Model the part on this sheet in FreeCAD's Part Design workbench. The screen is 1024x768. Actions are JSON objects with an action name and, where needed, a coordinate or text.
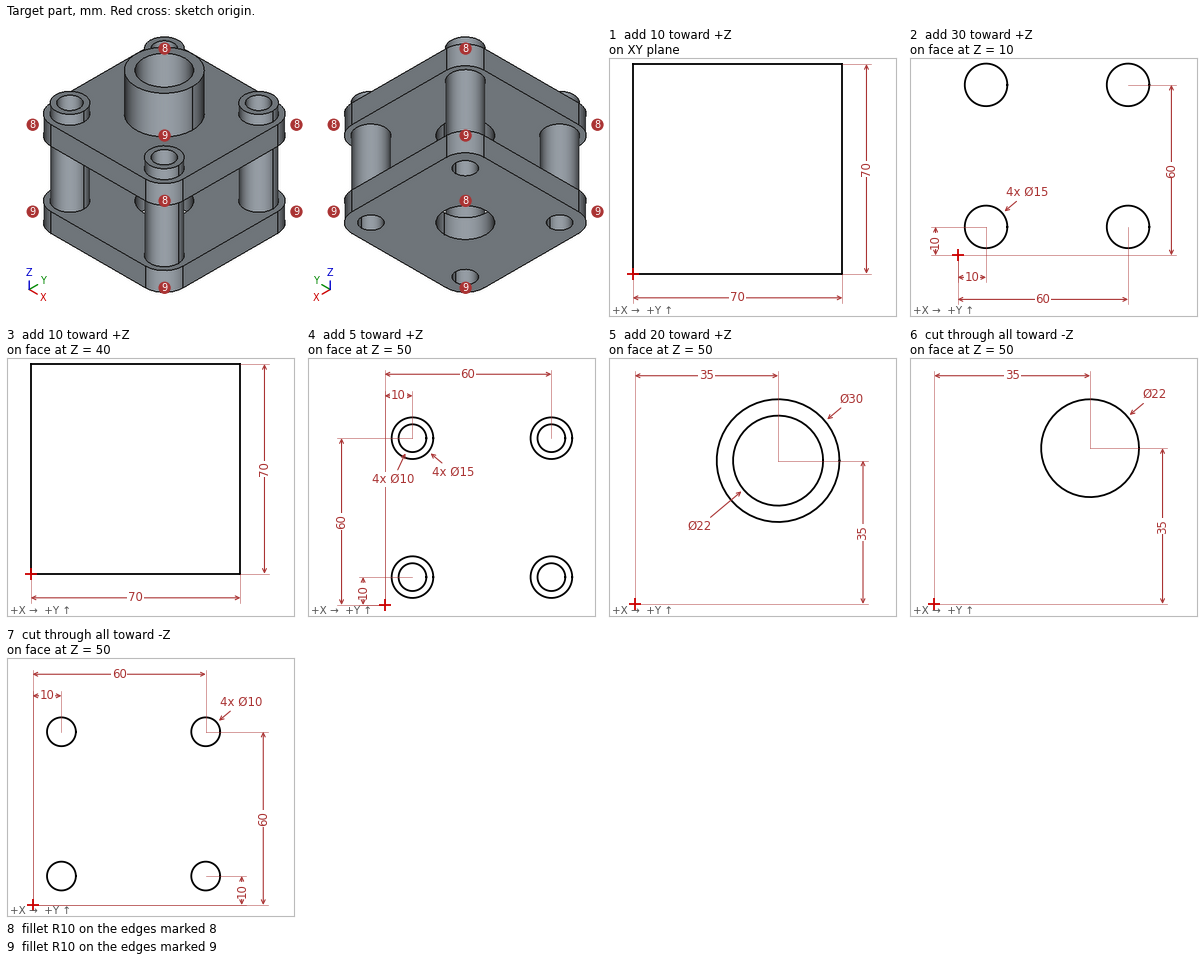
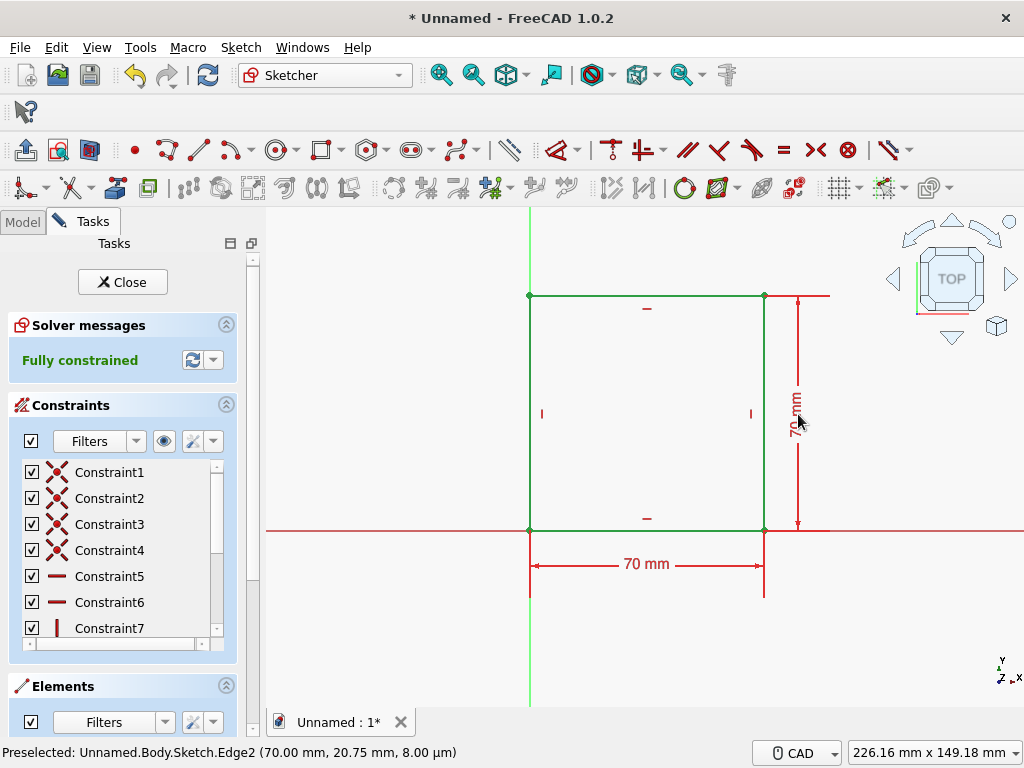
{"action": "left_click", "coordinate": [123, 282]}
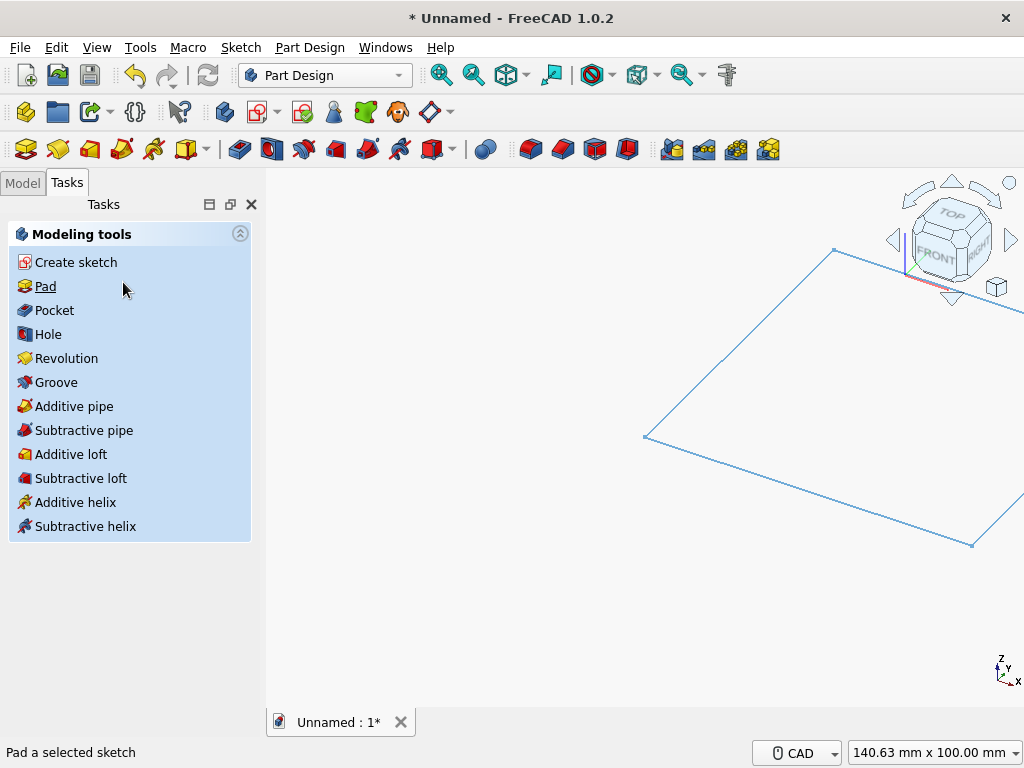
{"action": "left_click", "coordinate": [26, 150]}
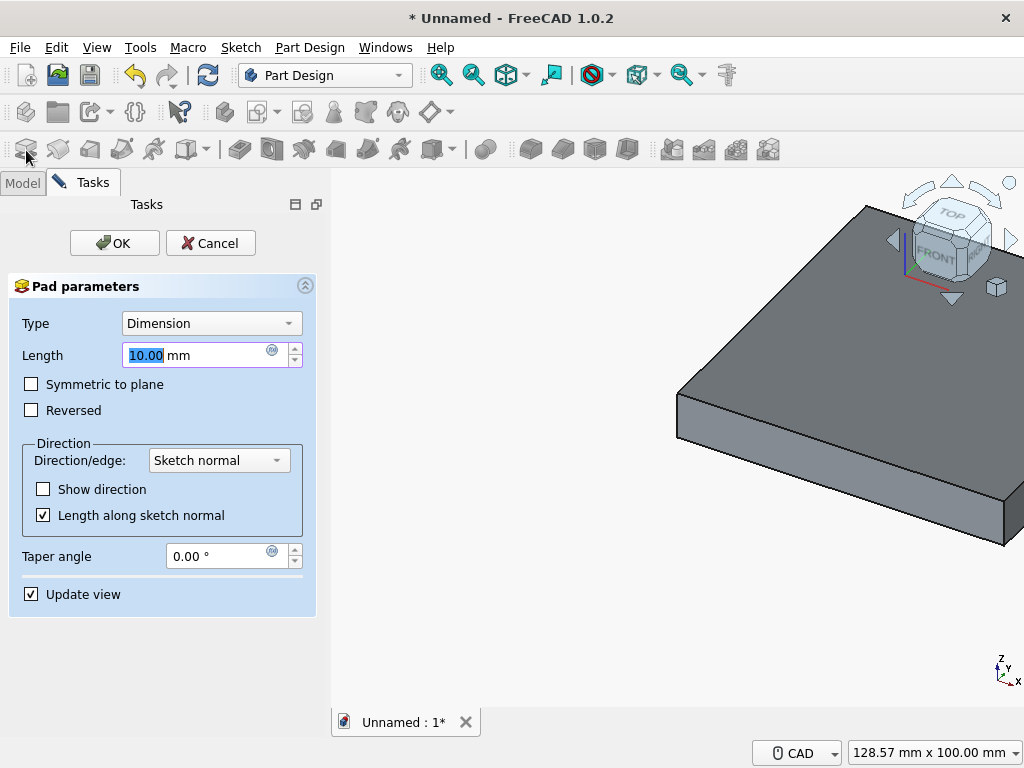
{"action": "type", "text": "10"}
{"action": "key", "text": "Tab"}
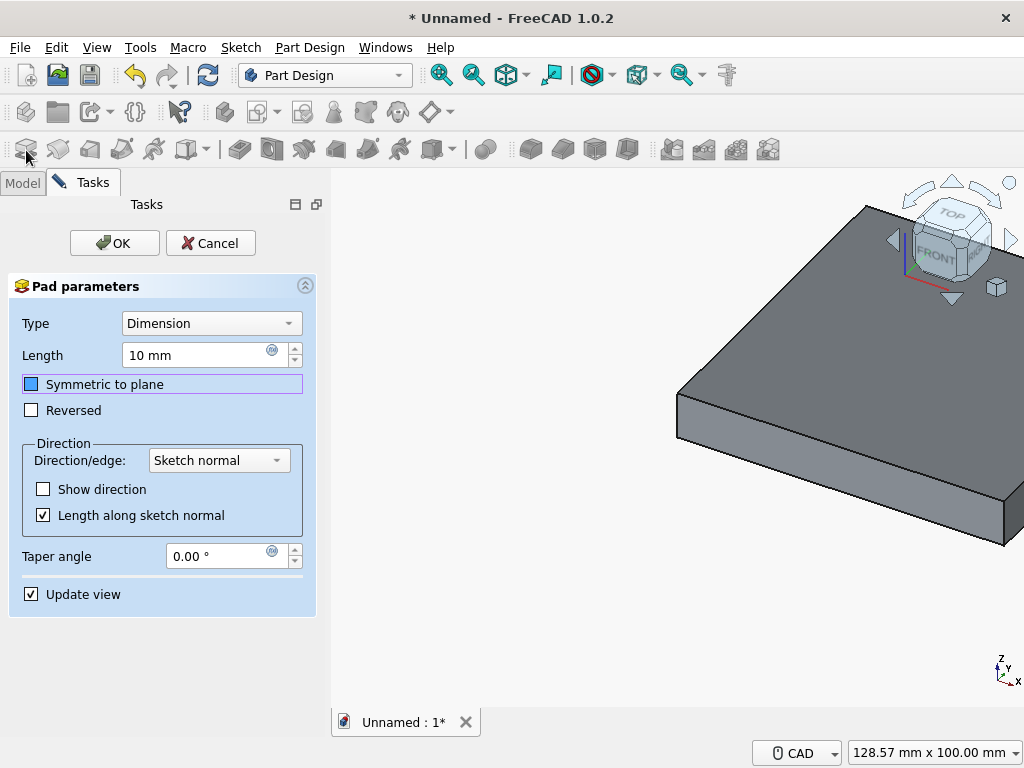
{"action": "left_click", "coordinate": [115, 243]}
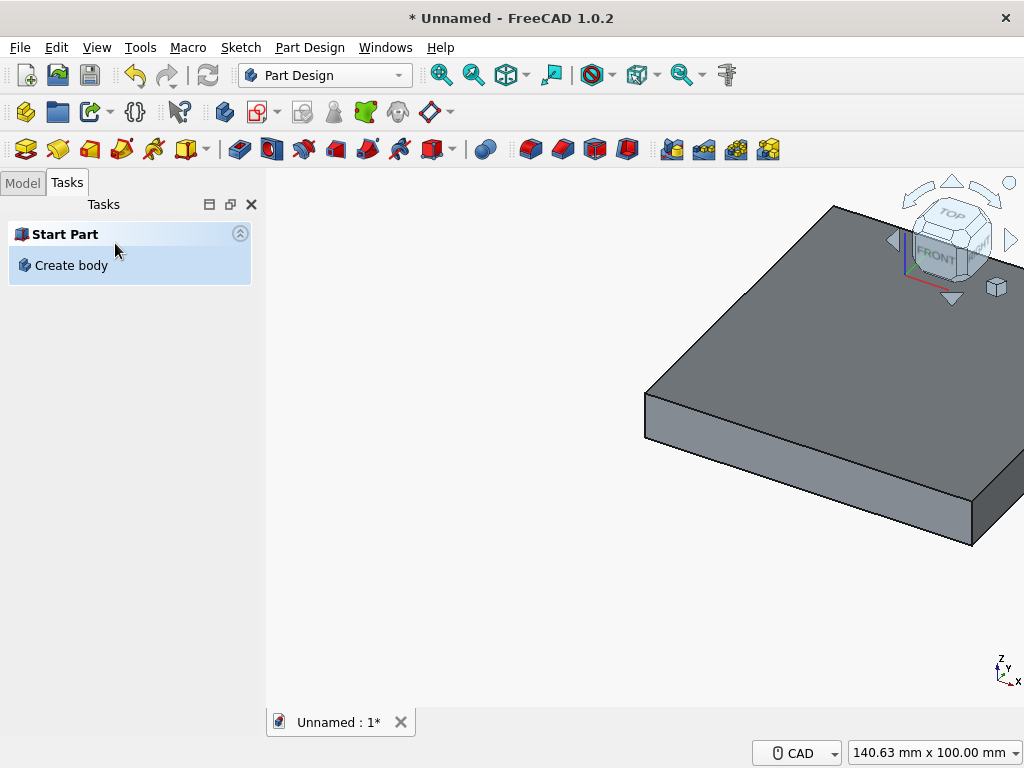
{"action": "key", "text": "v f"}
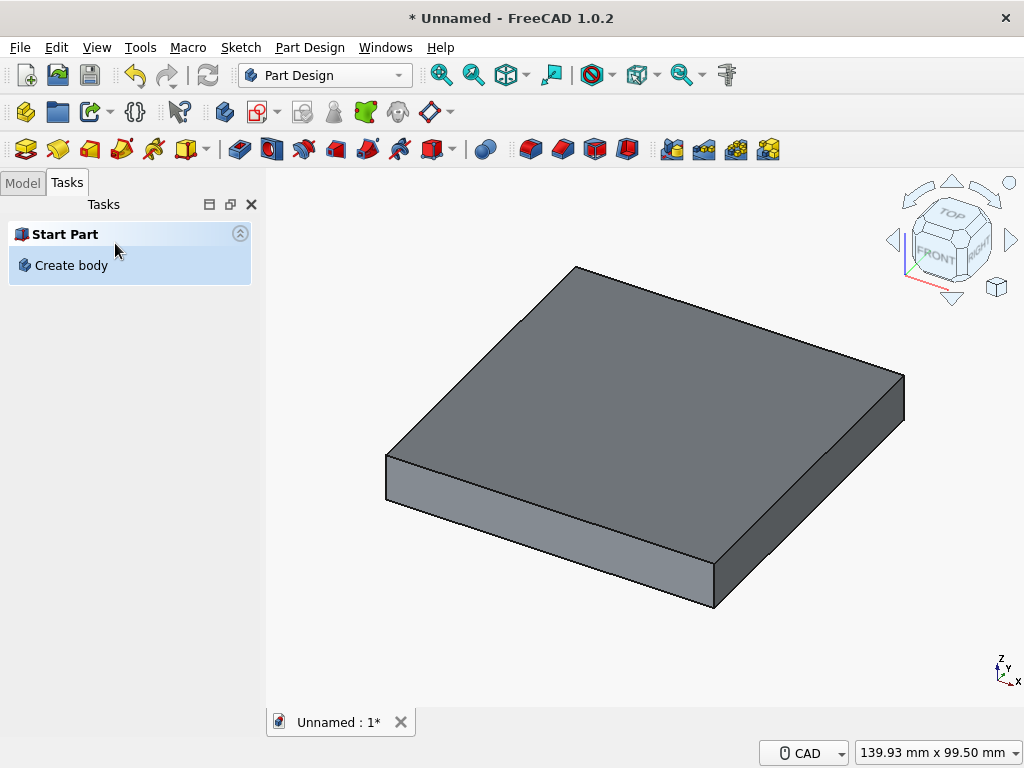
{"action": "left_click", "coordinate": [645, 414]}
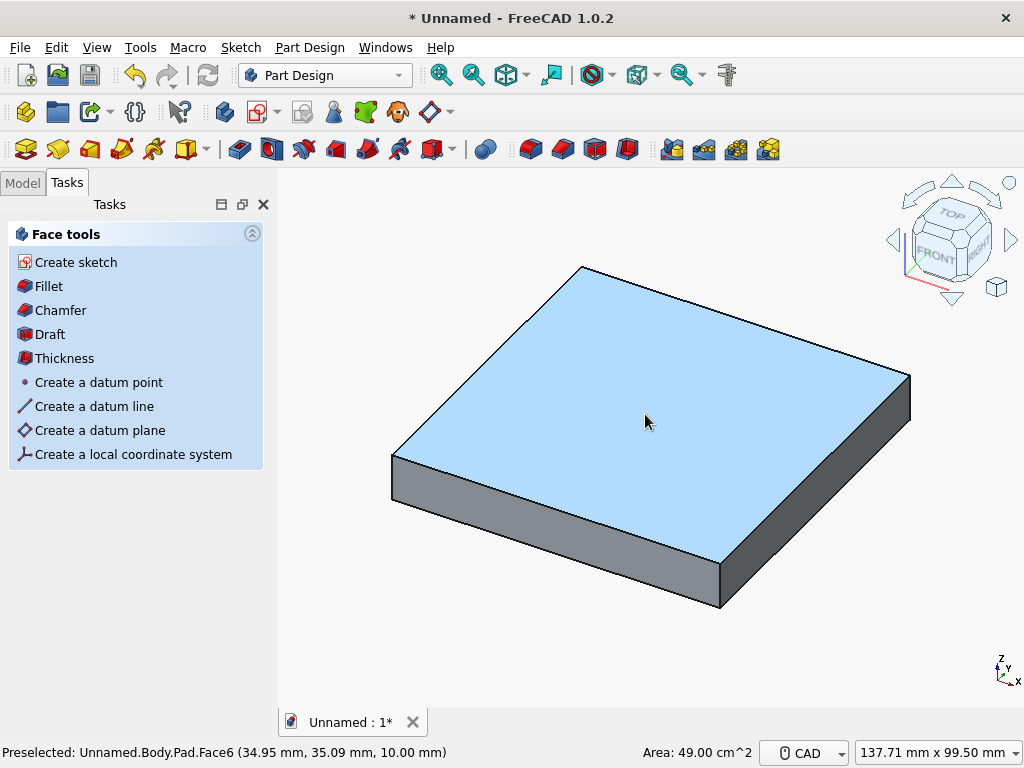
{"action": "left_click", "coordinate": [258, 112]}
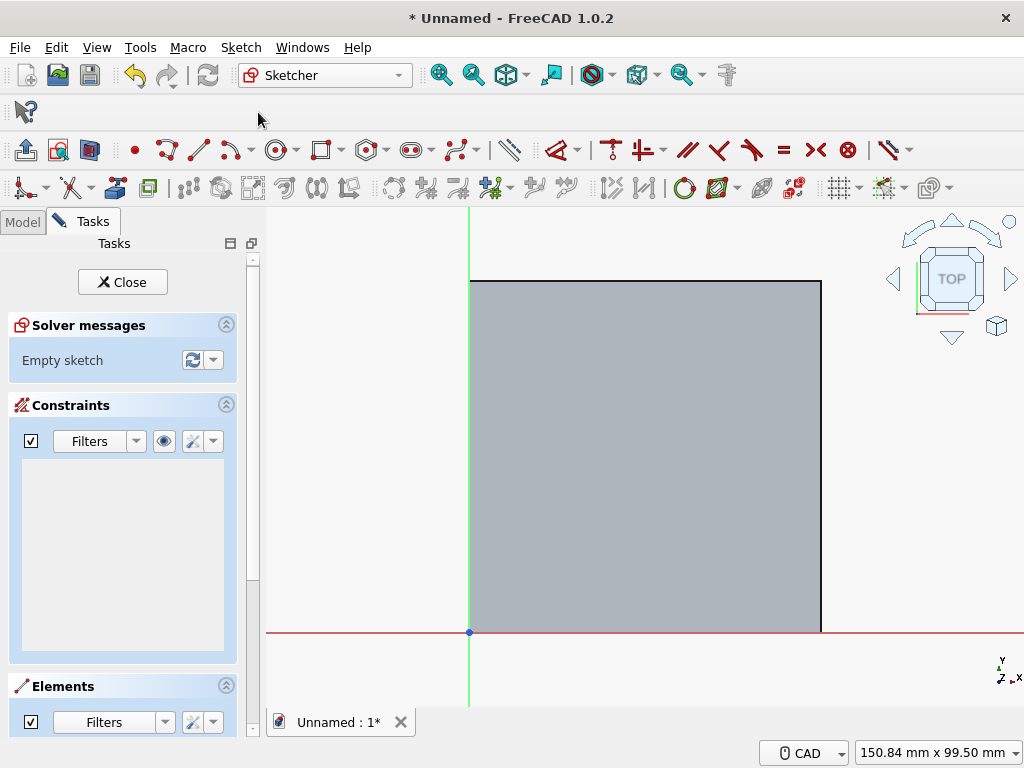
{"action": "left_click", "coordinate": [276, 150]}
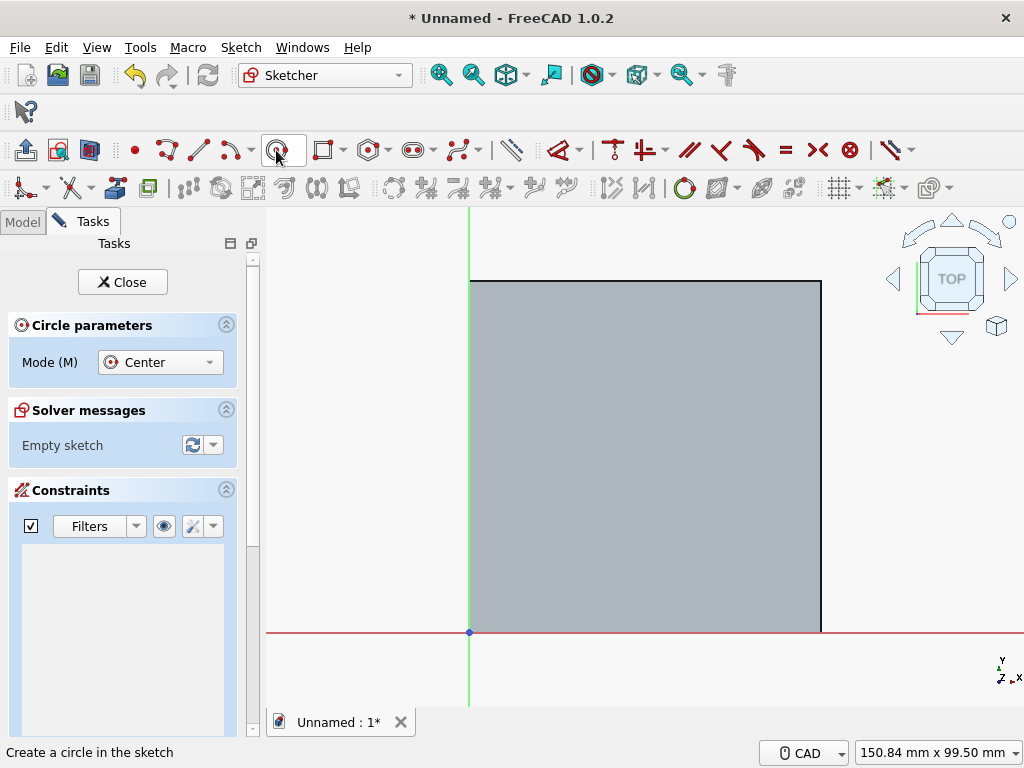
{"action": "left_click", "coordinate": [519, 583]}
{"action": "left_click", "coordinate": [546, 556]}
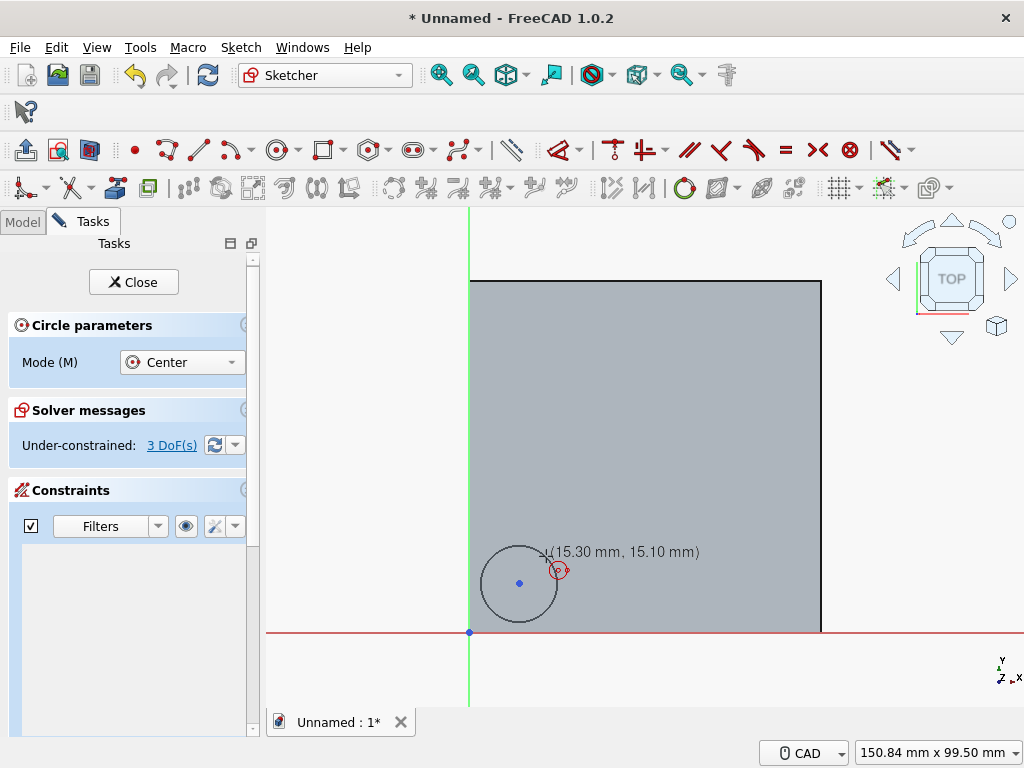
{"action": "left_click", "coordinate": [771, 583]}
{"action": "left_click", "coordinate": [797, 556]}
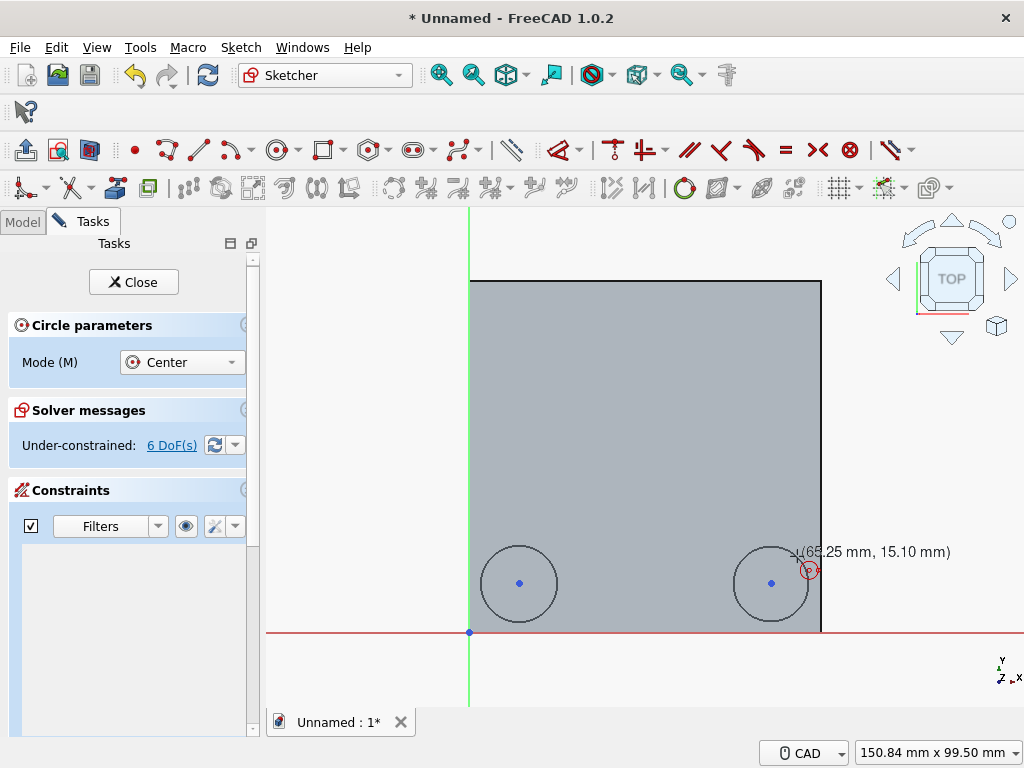
{"action": "left_click", "coordinate": [771, 331]}
{"action": "left_click", "coordinate": [797, 305]}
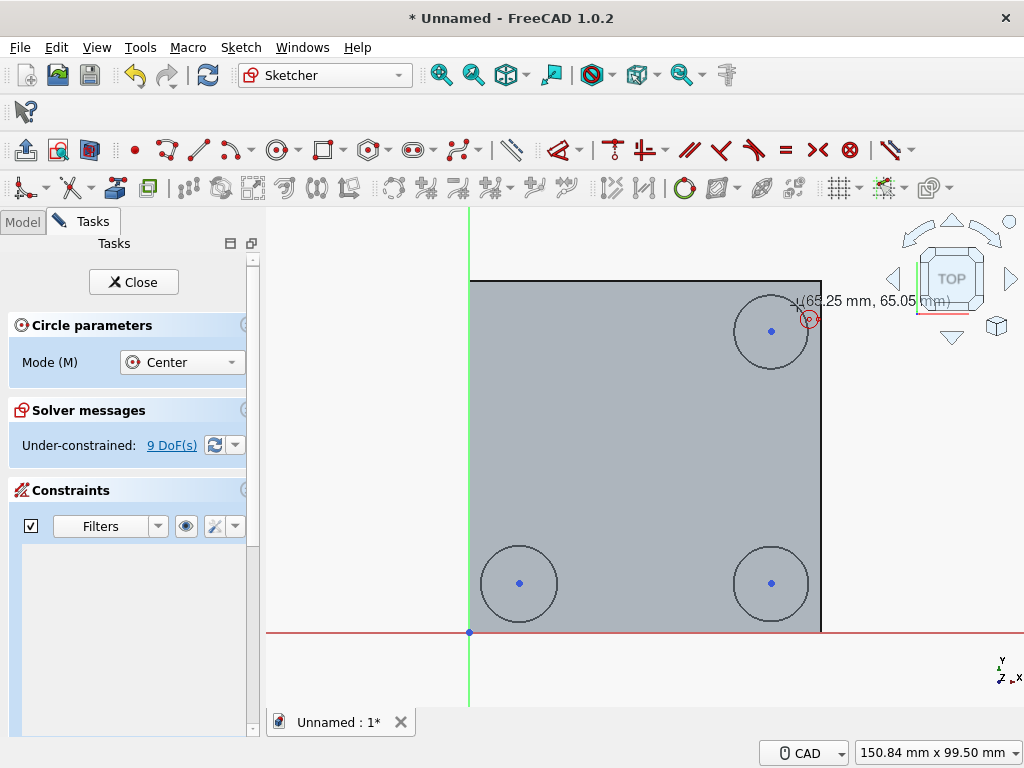
{"action": "left_click", "coordinate": [519, 331]}
{"action": "left_click", "coordinate": [546, 305]}
{"action": "key", "text": "Escape"}